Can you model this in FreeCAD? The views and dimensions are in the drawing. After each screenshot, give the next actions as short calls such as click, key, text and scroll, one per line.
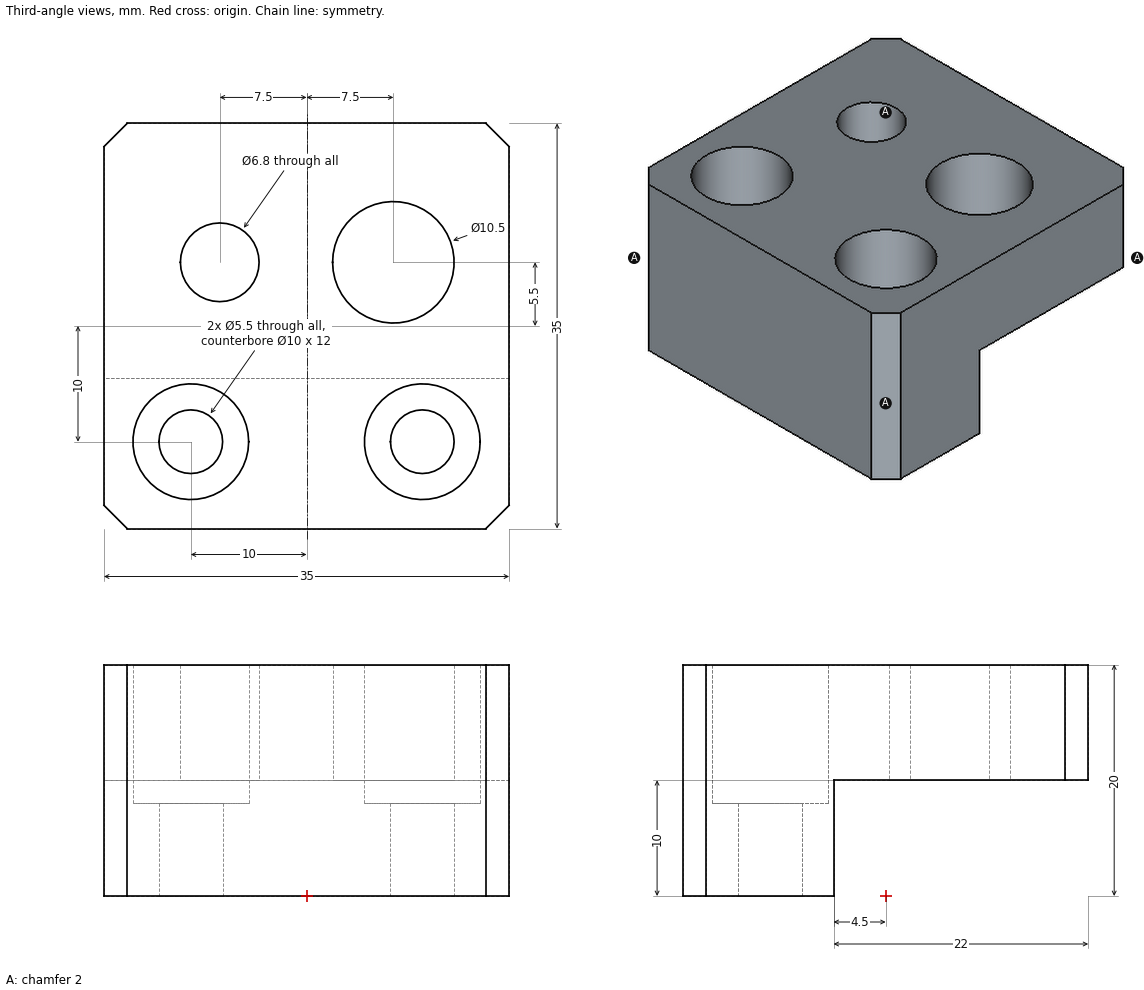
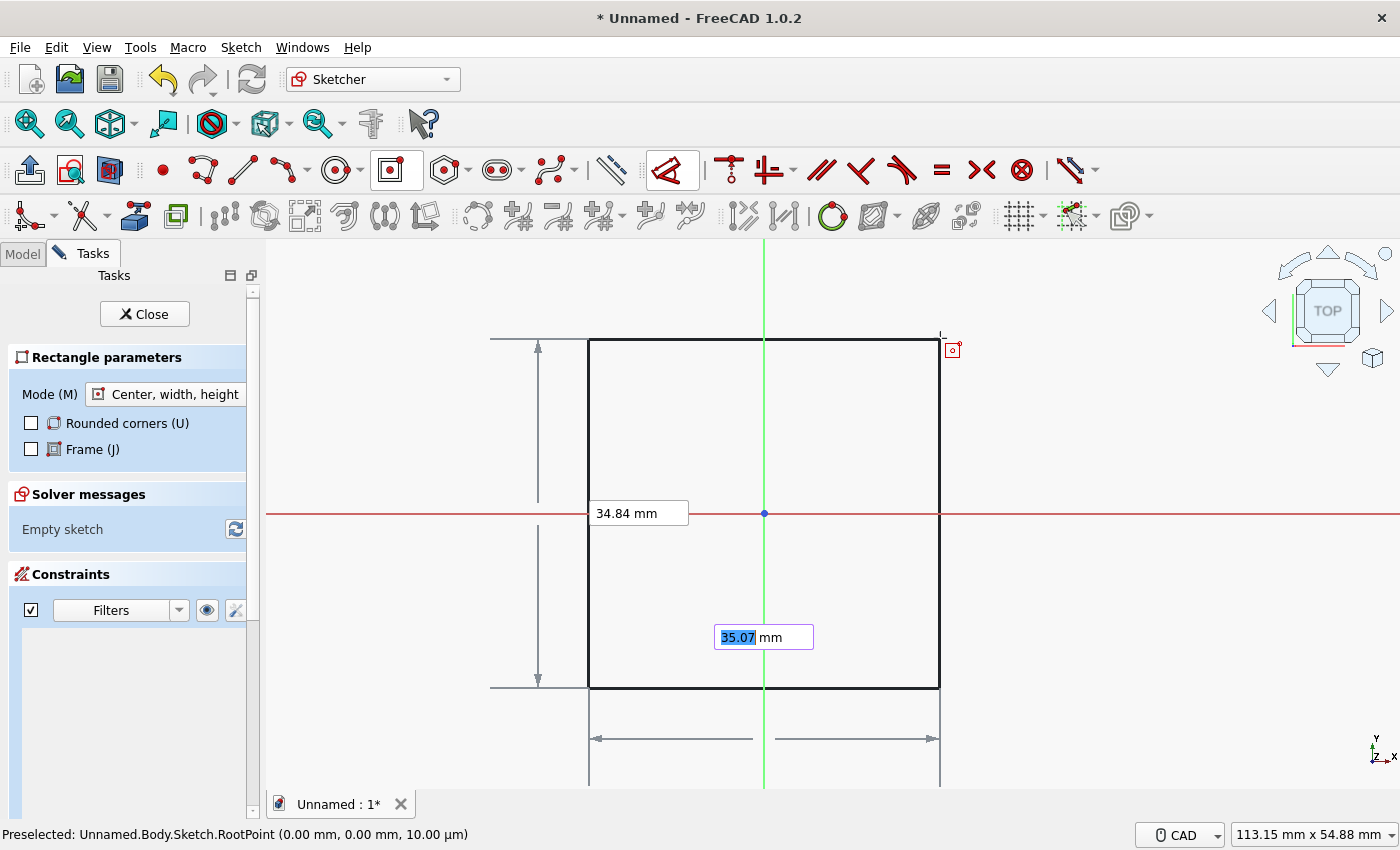
text(35)
key(Tab)
text(35)
key(Return)
key(Escape)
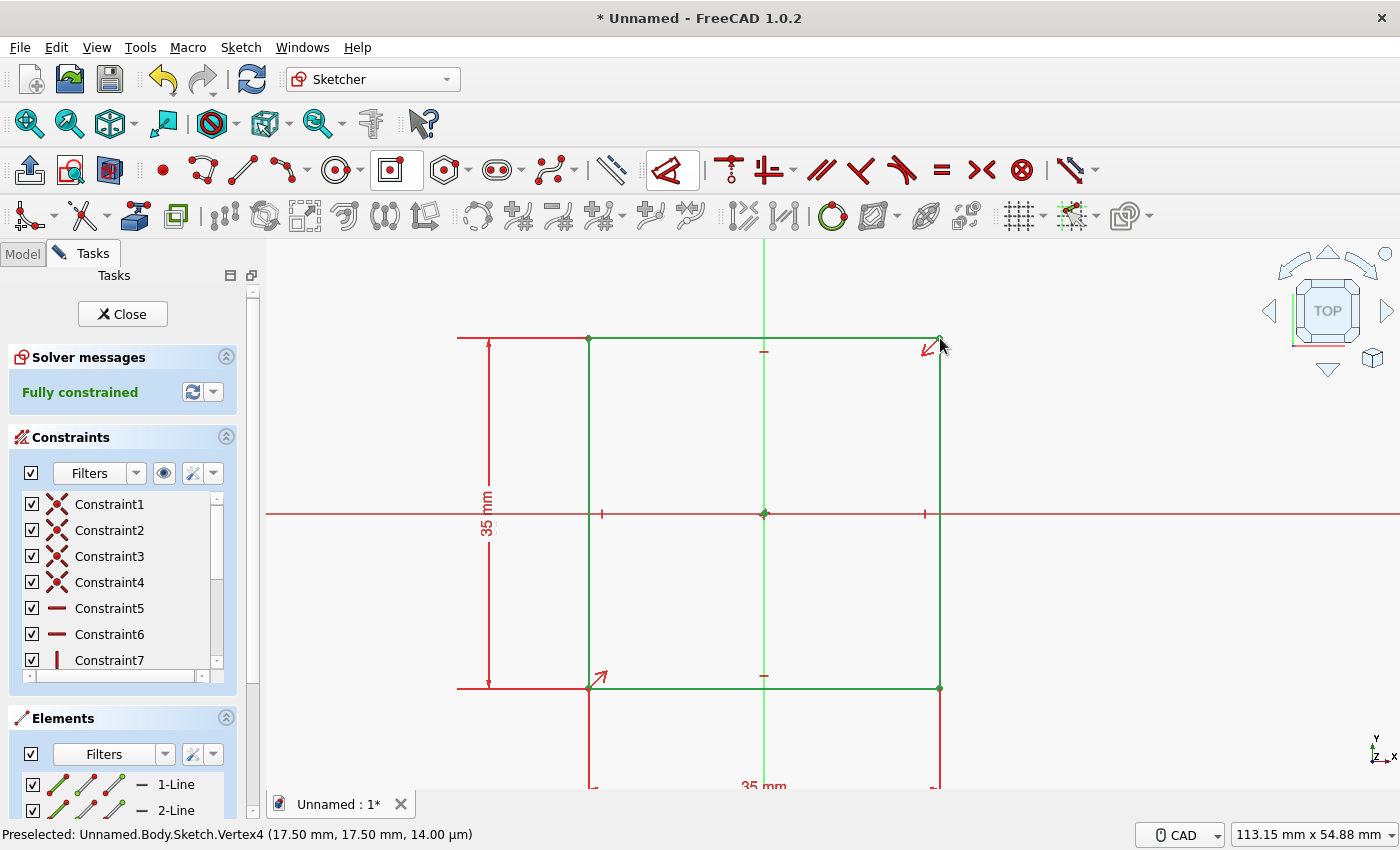
click(123, 314)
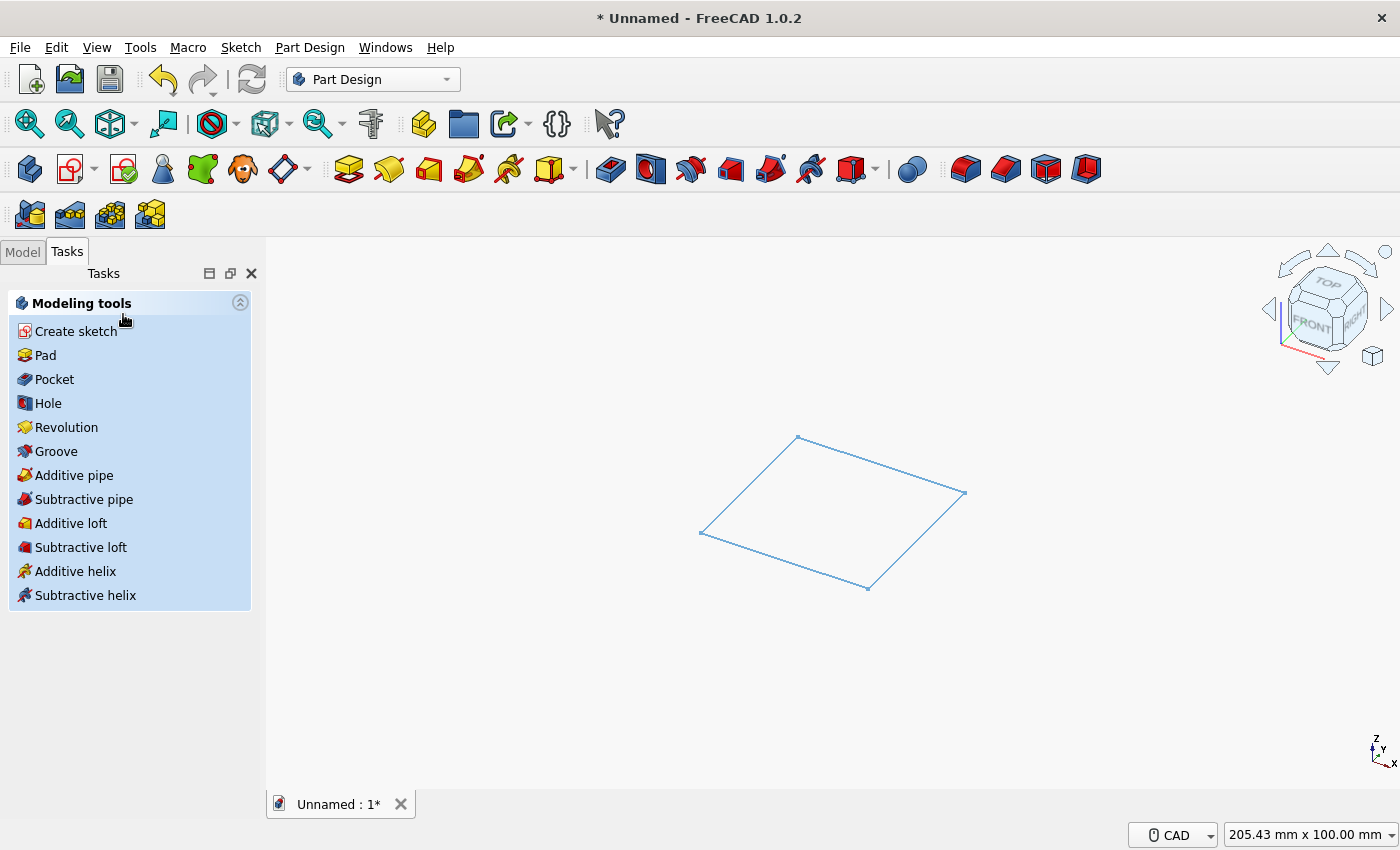
click(350, 170)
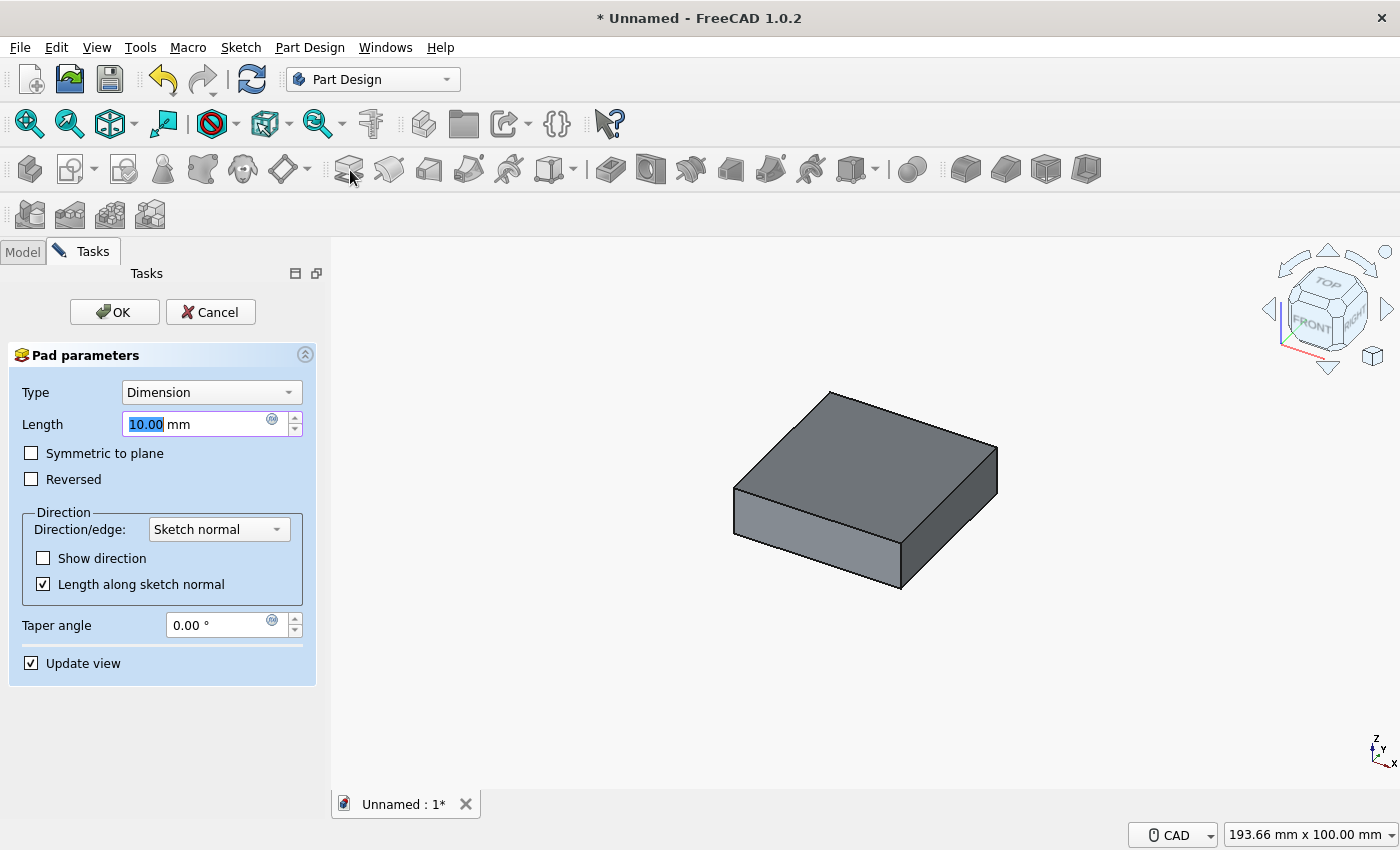
text(20)
key(Tab)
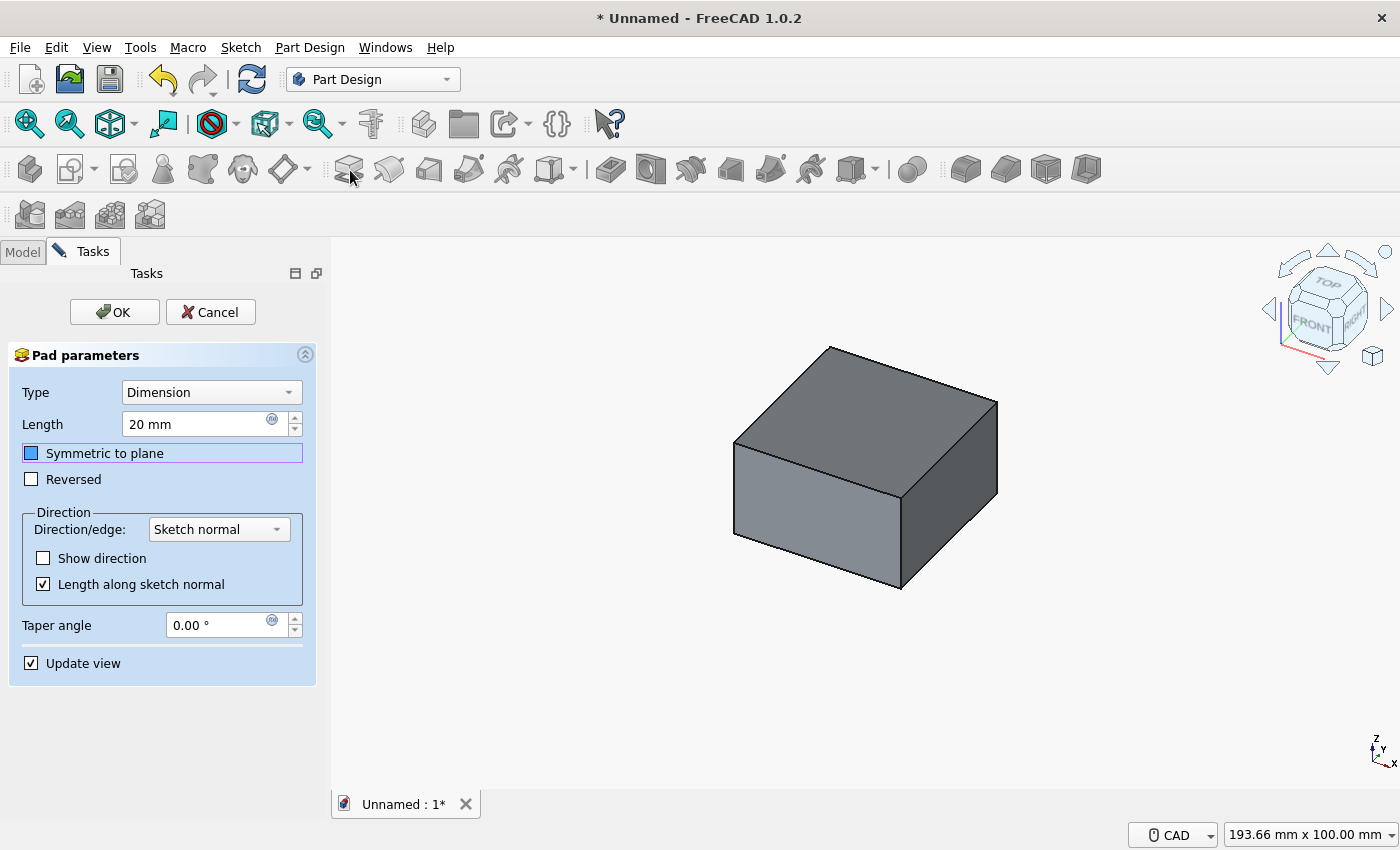
click(115, 312)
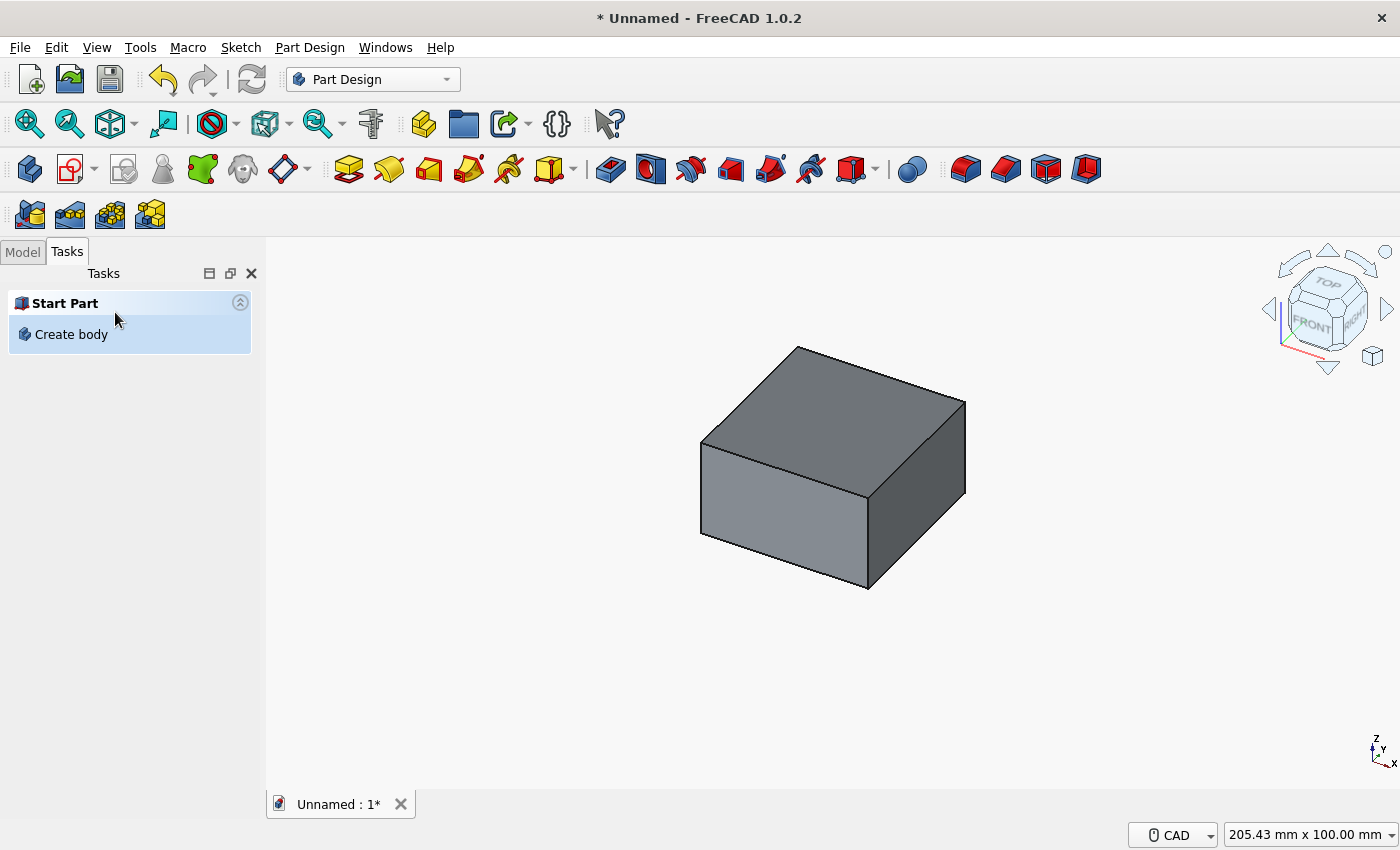
click(30, 124)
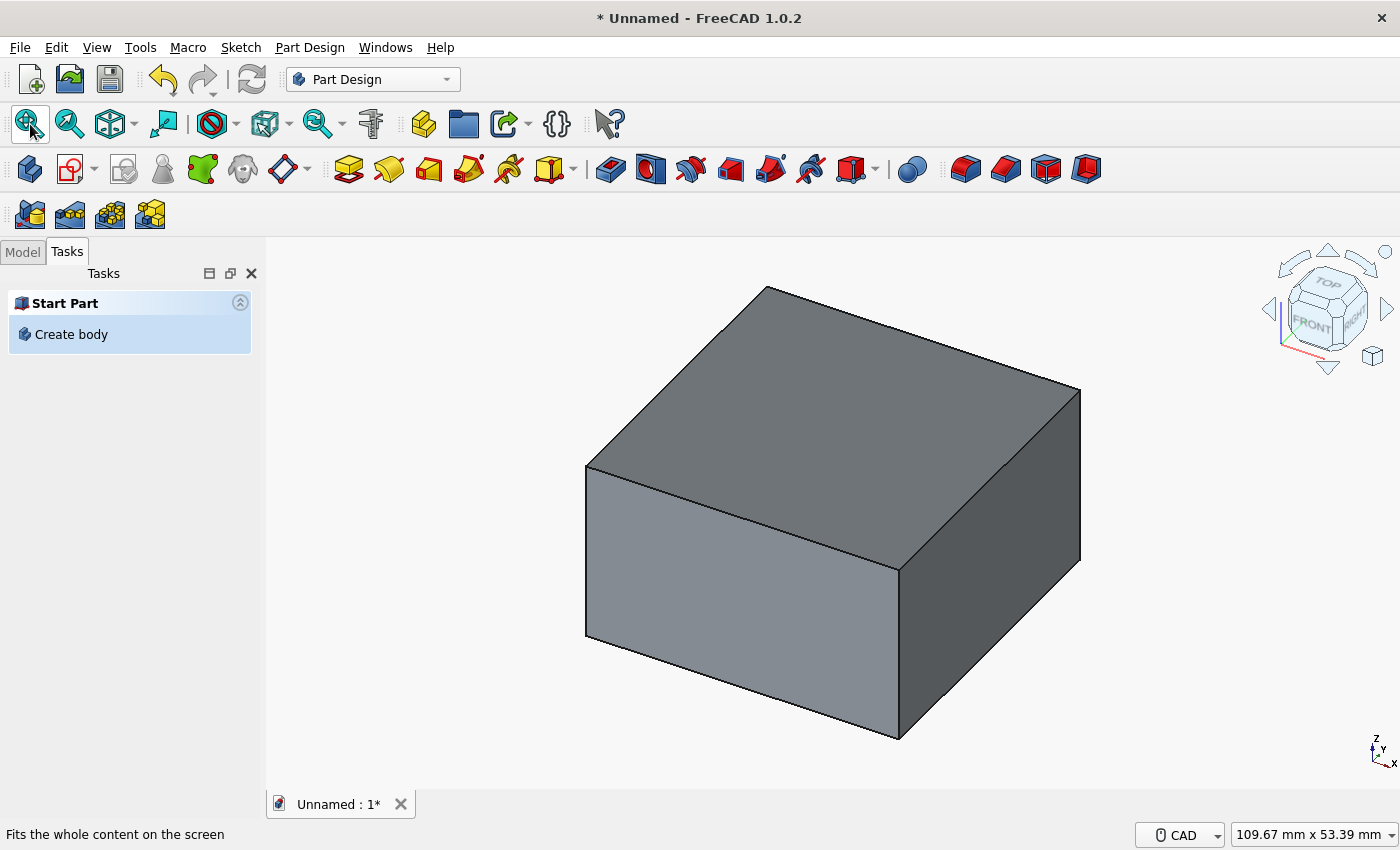
click(899, 654)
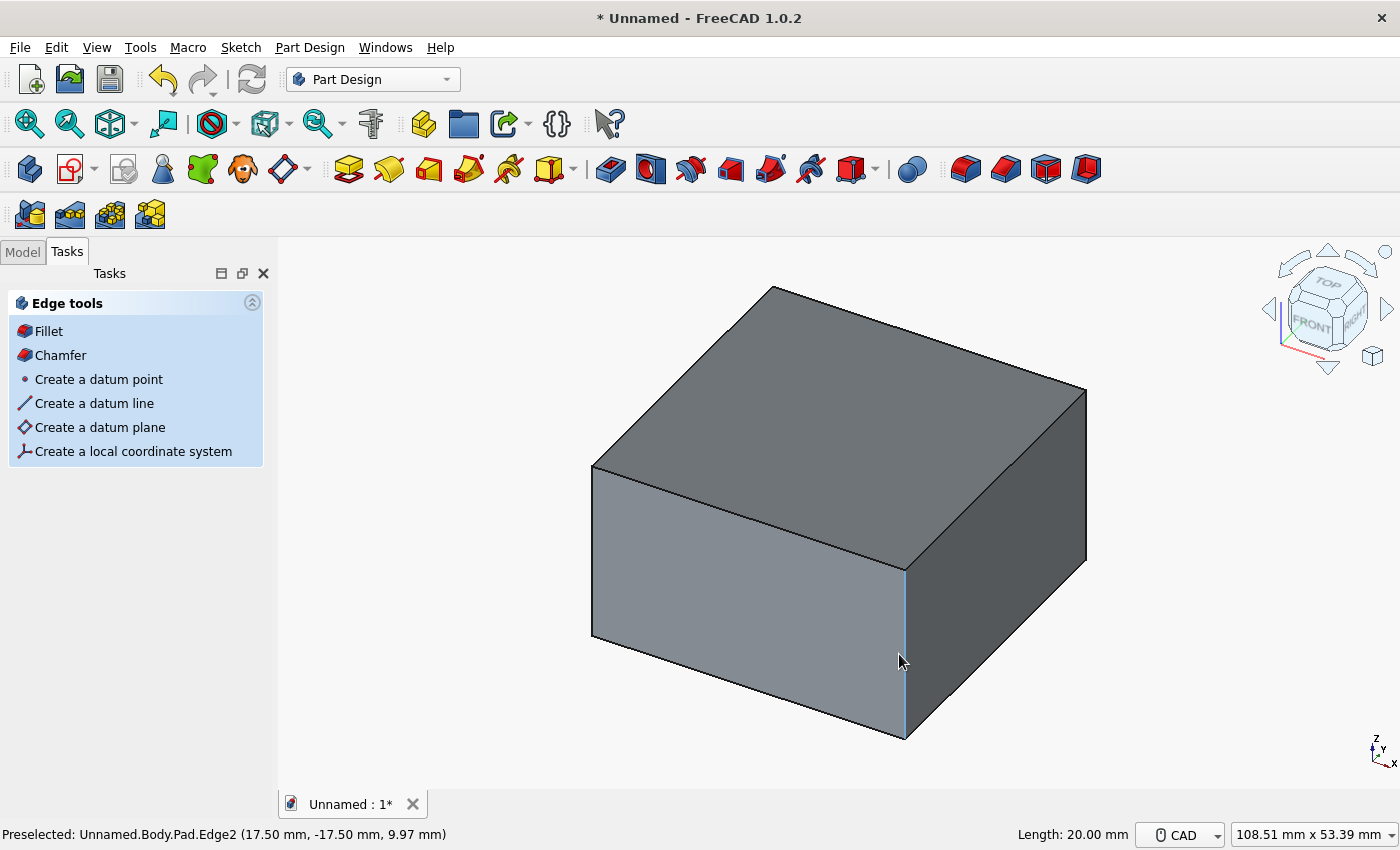
key(0)